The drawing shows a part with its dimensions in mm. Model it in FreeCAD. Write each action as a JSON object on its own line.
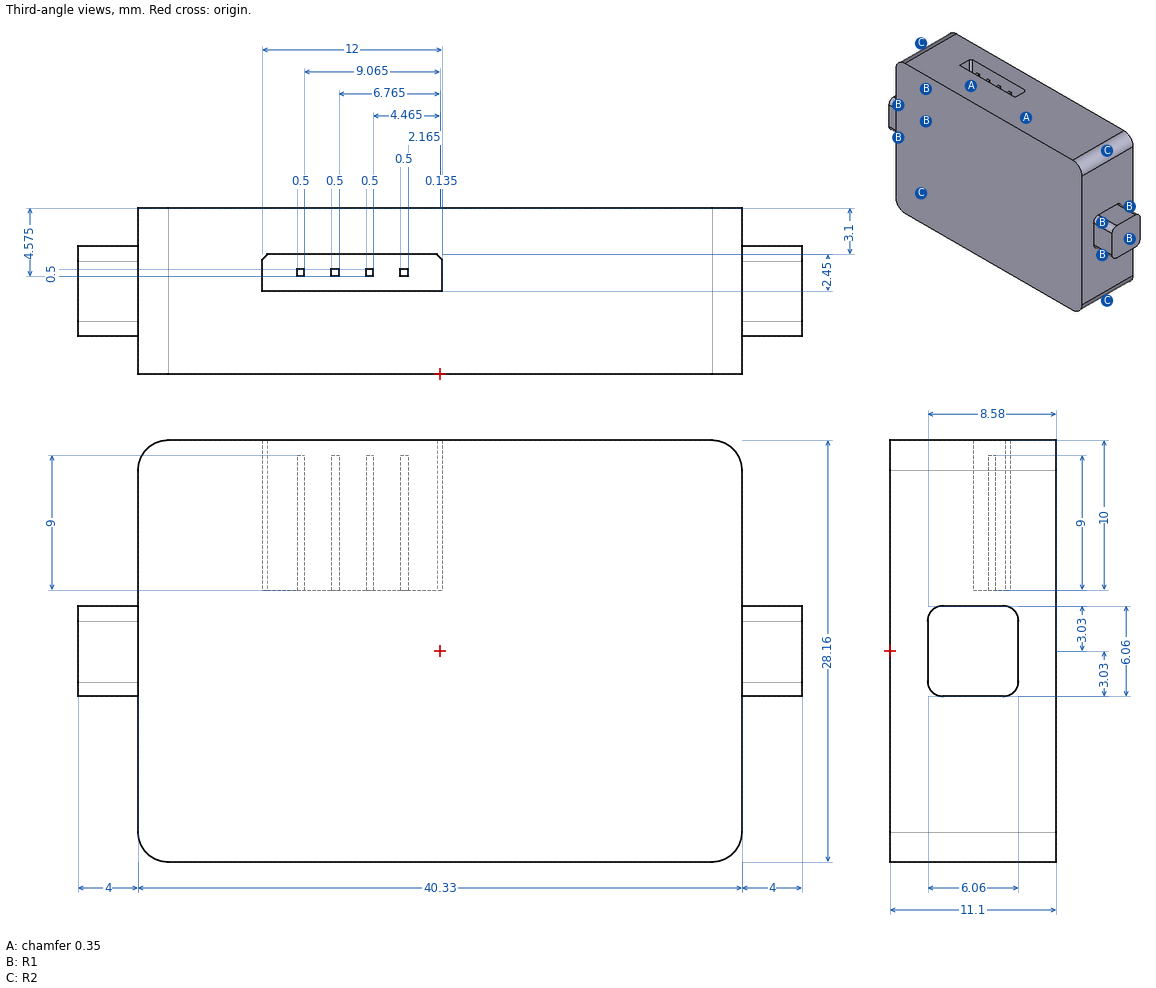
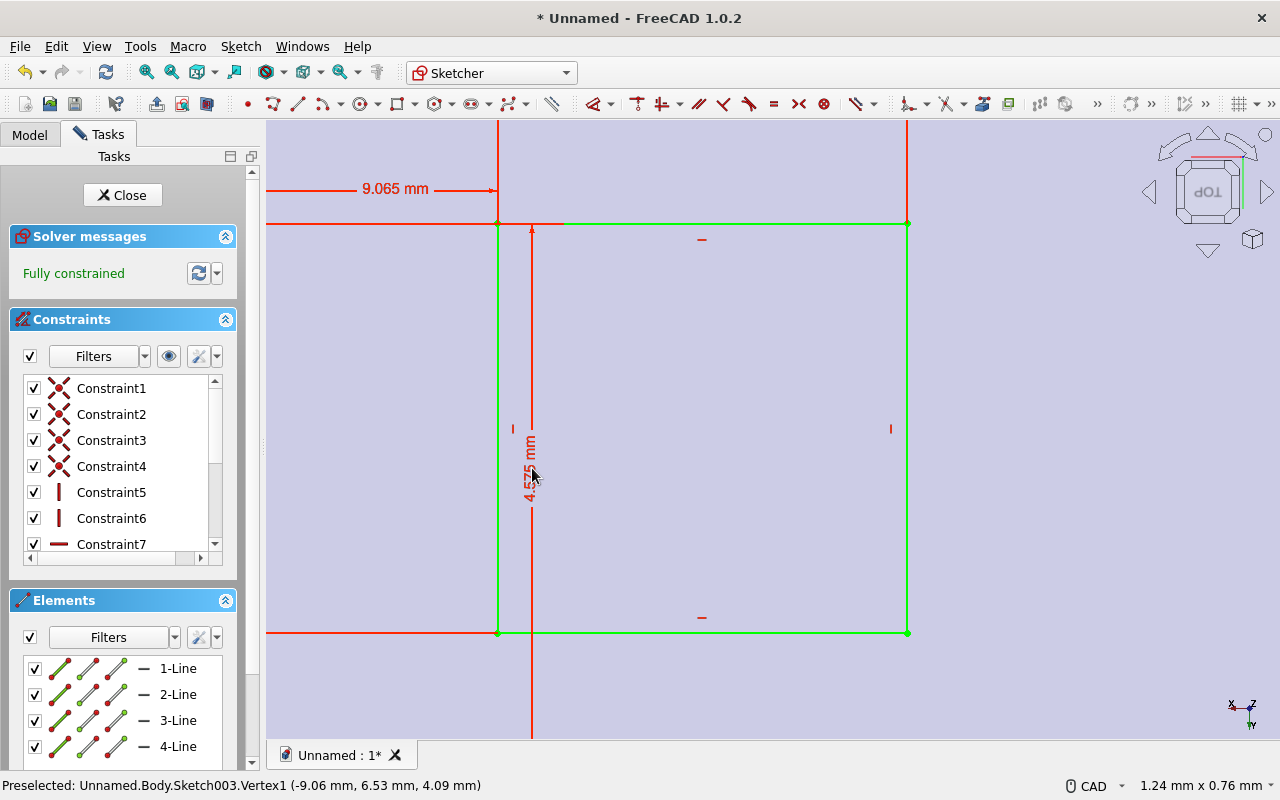
{"action": "left_click", "coordinate": [123, 195]}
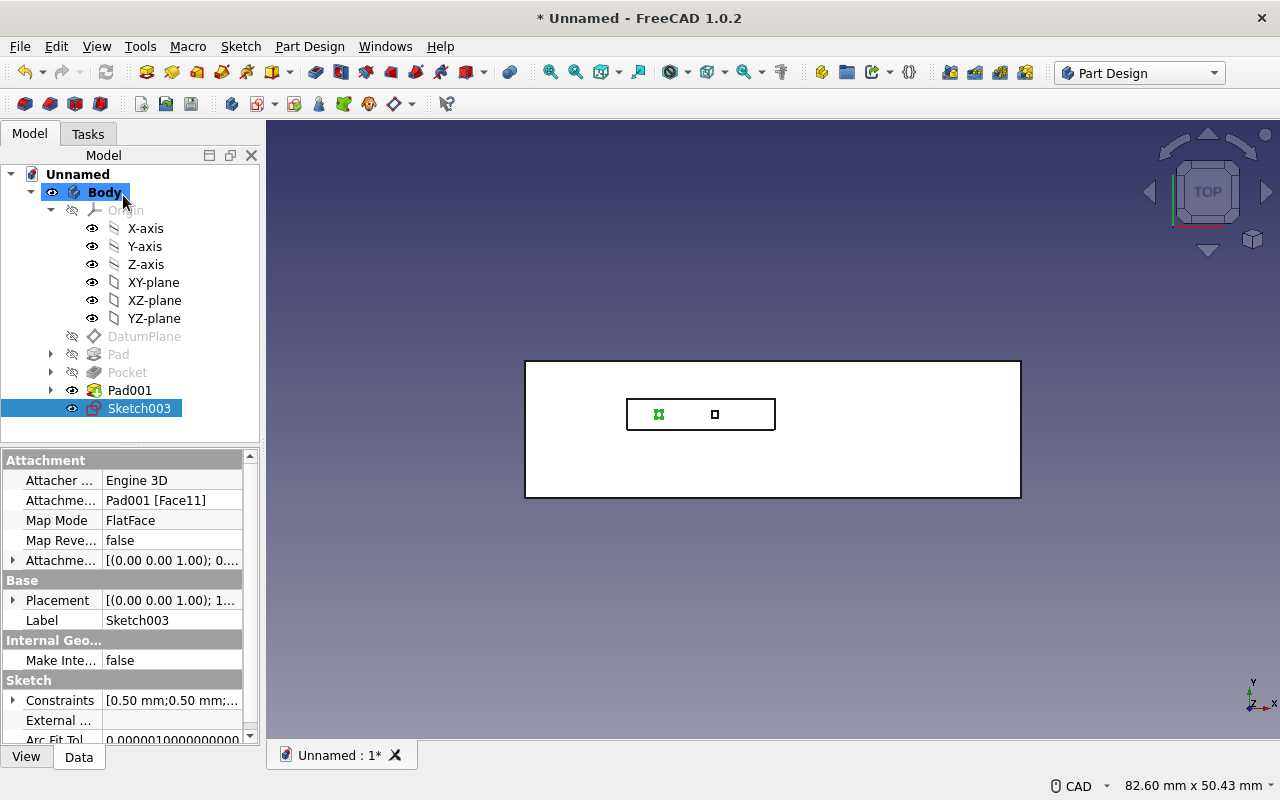
{"action": "left_click", "coordinate": [147, 72]}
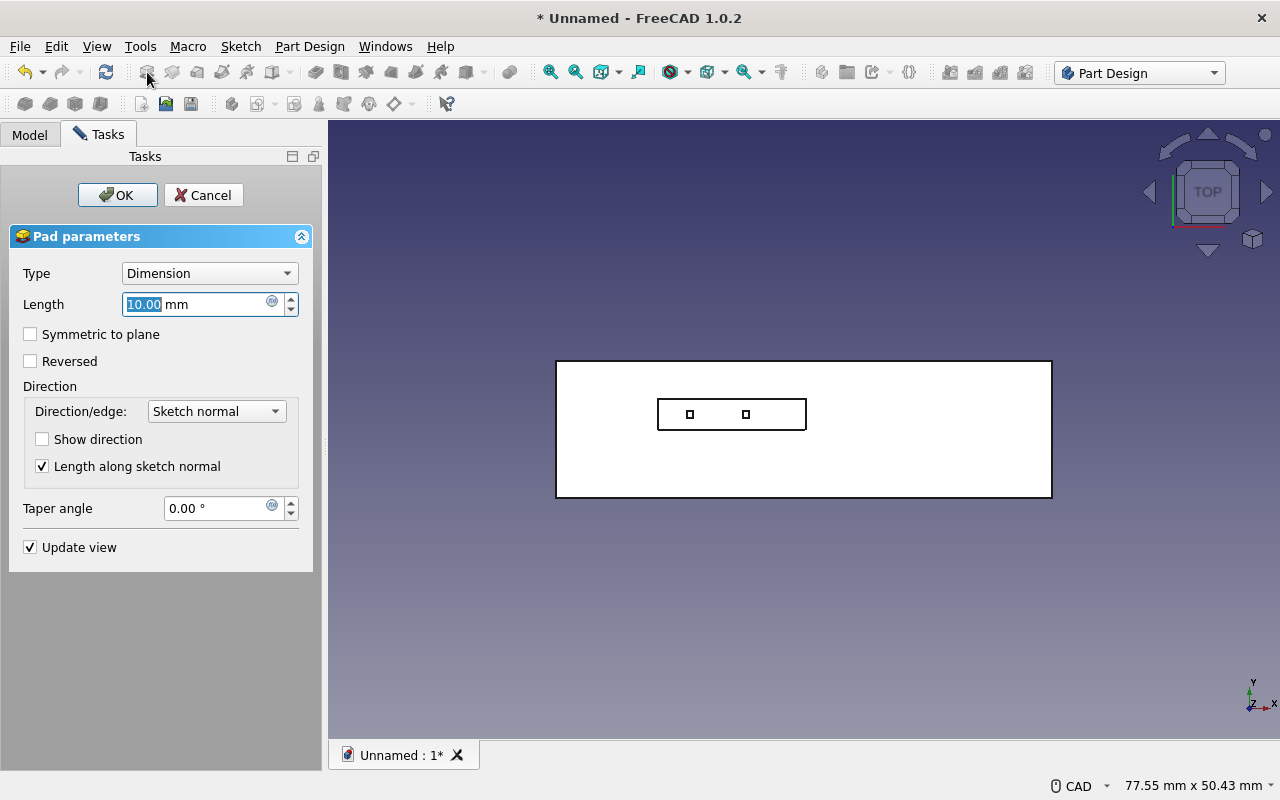
{"action": "type", "text": "9"}
{"action": "key", "text": "Tab"}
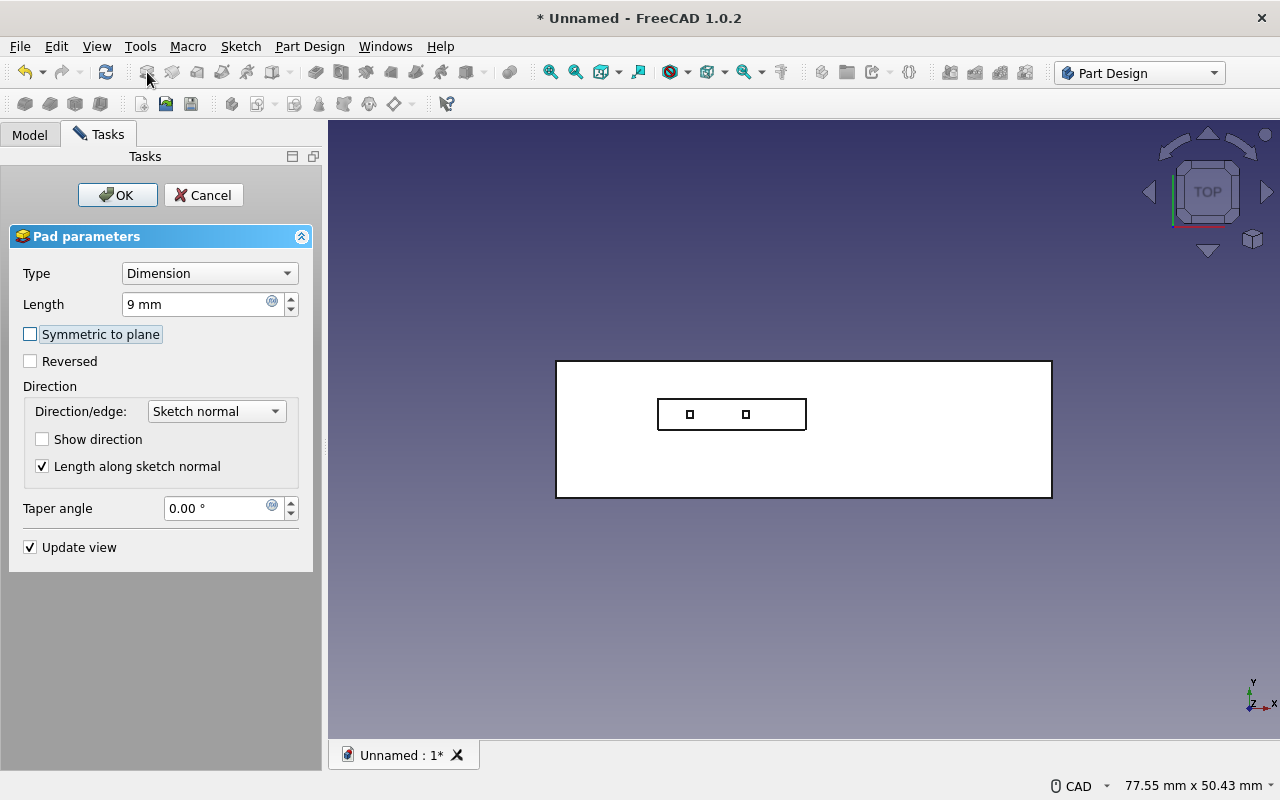
{"action": "left_click", "coordinate": [118, 195]}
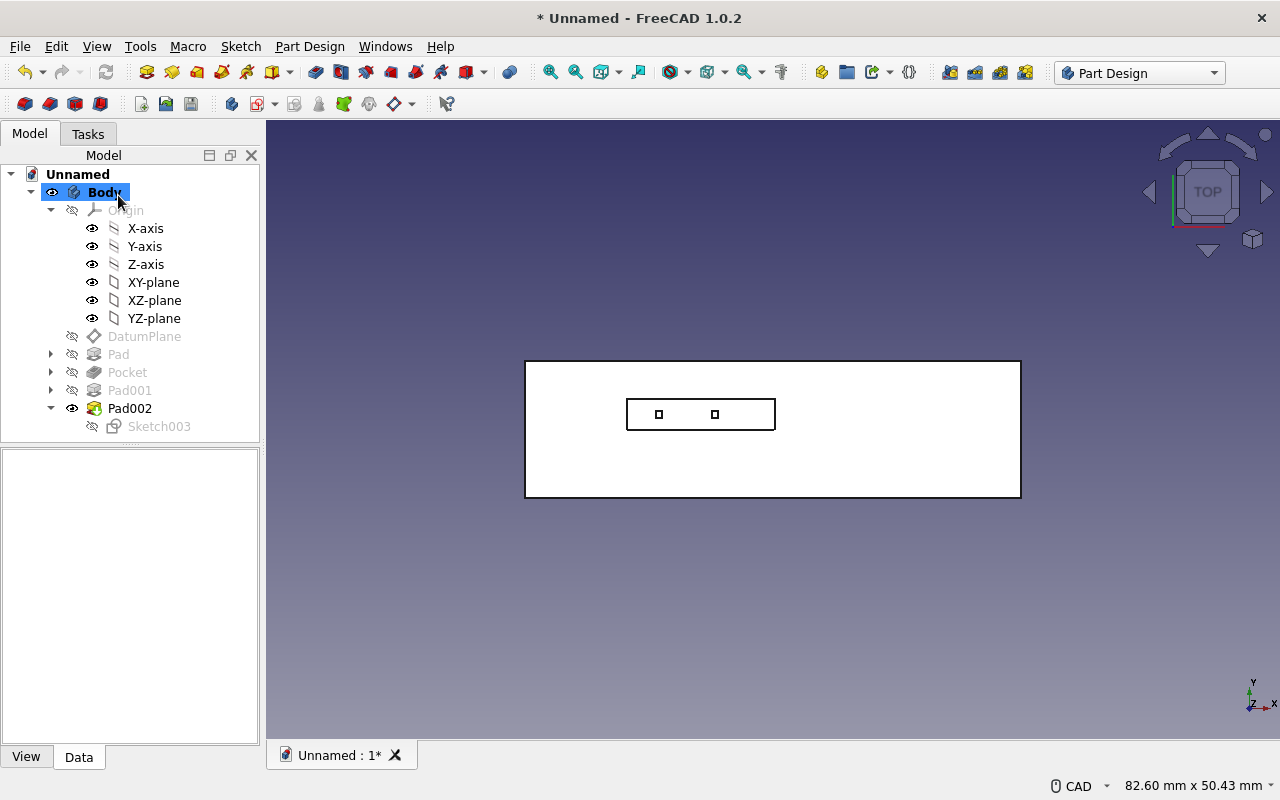
{"action": "left_click", "coordinate": [743, 413]}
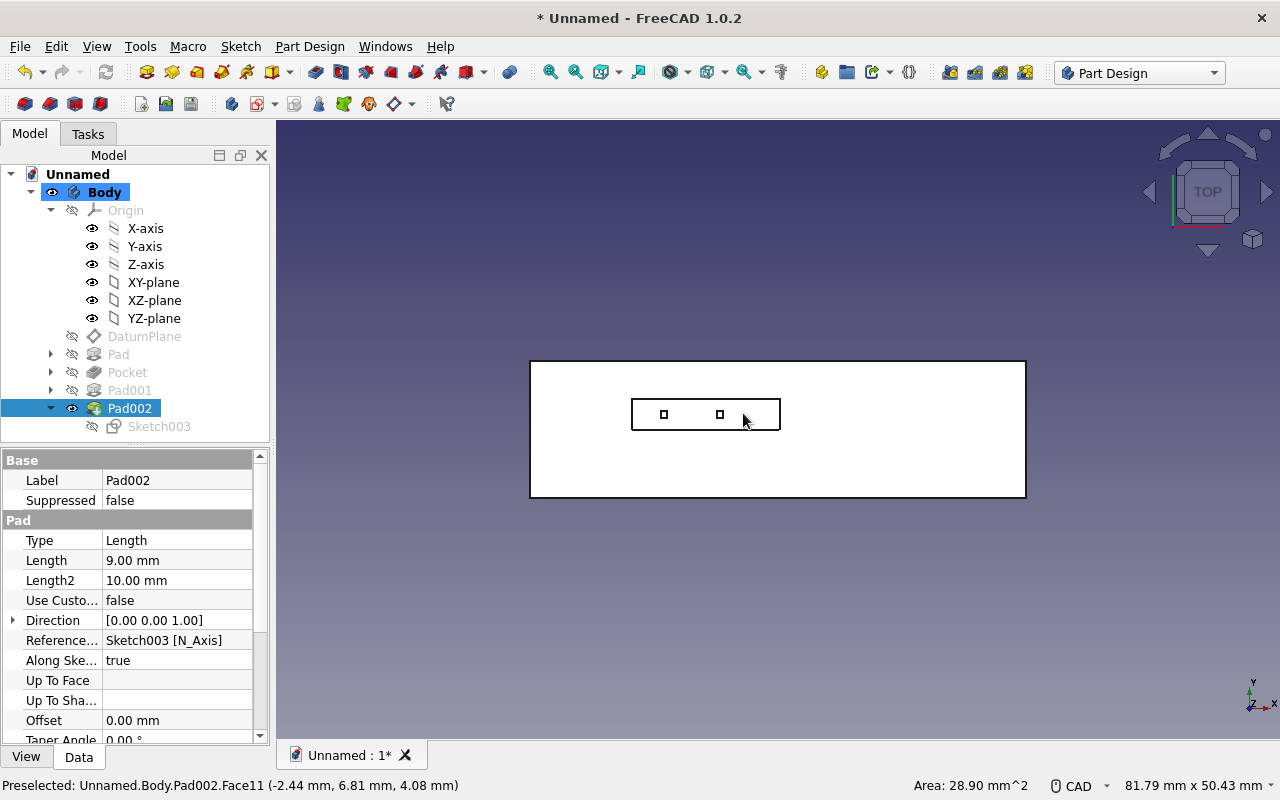
{"action": "left_click", "coordinate": [256, 104]}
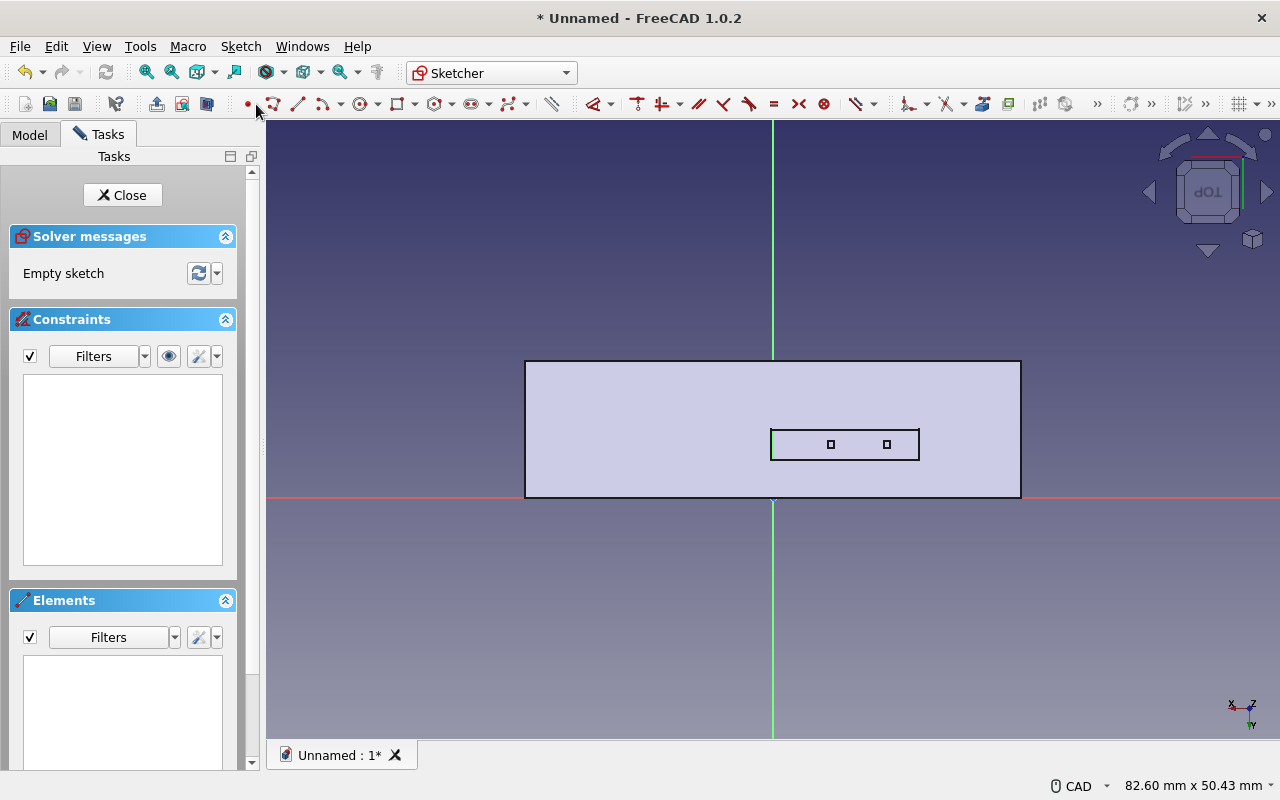
{"action": "left_click", "coordinate": [207, 104]}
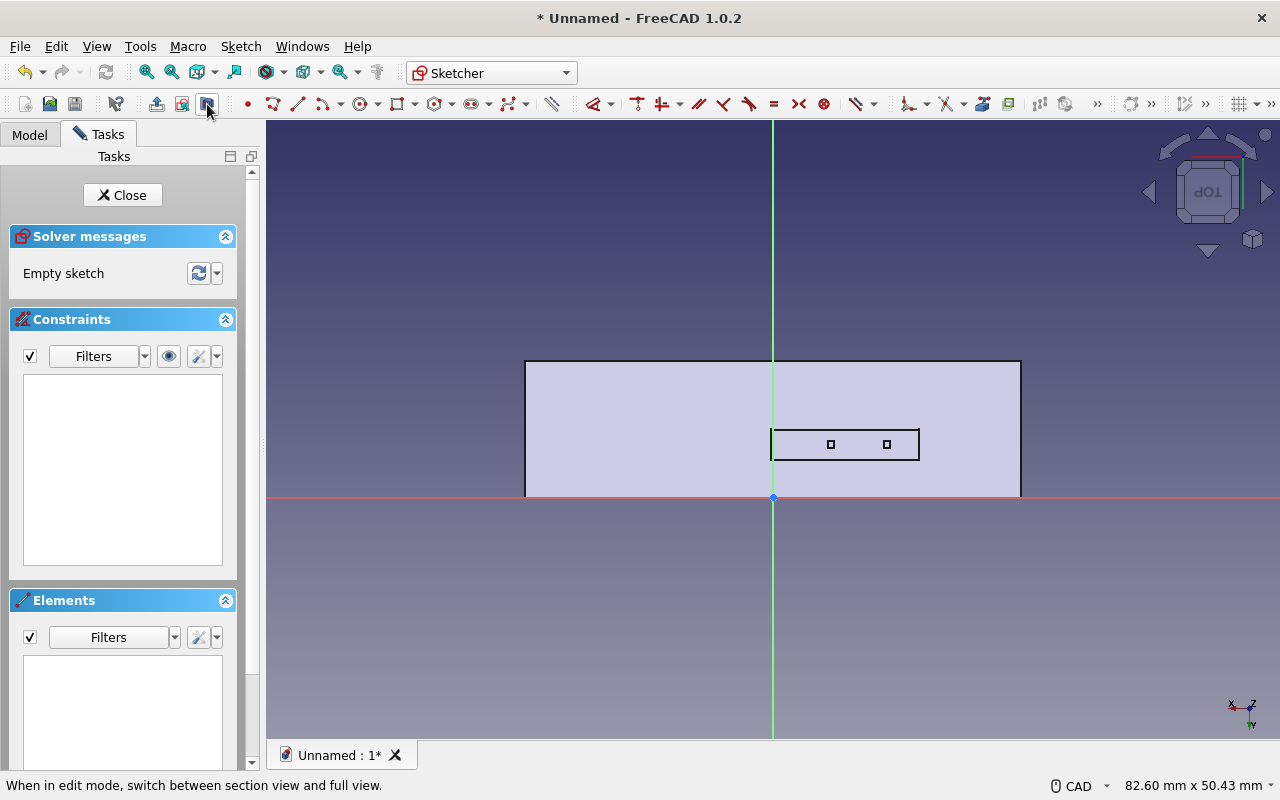
{"action": "scroll", "coordinate": [867, 445], "scroll_direction": "up", "scroll_amount": 15}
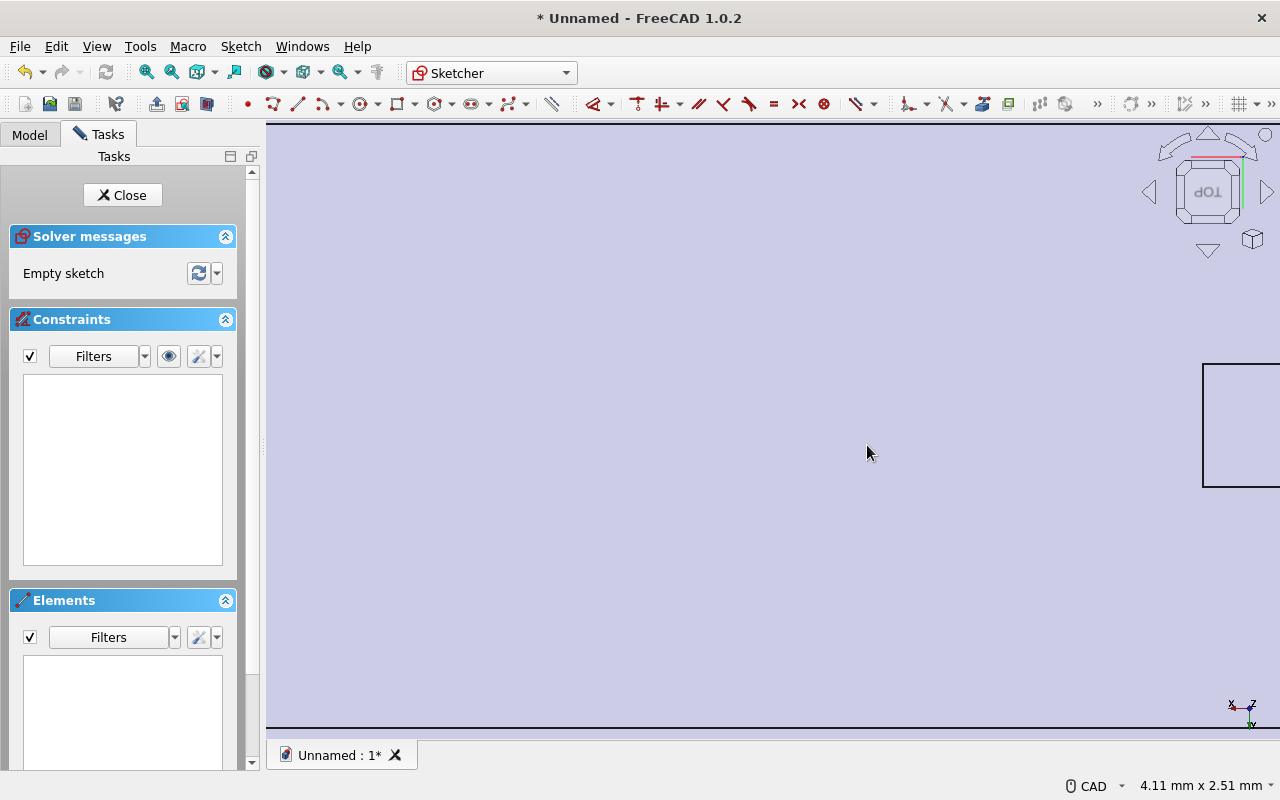
{"action": "scroll", "coordinate": [694, 424], "scroll_direction": "up", "scroll_amount": 6}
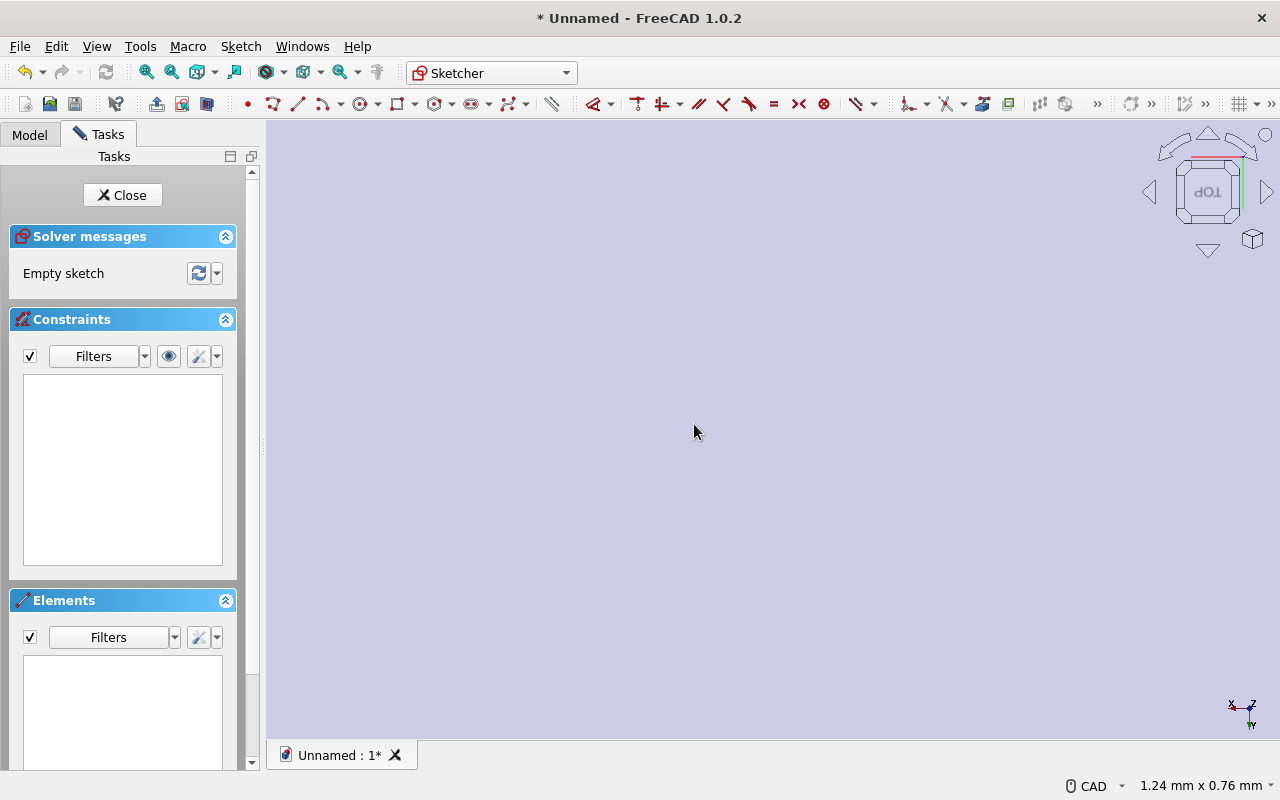
{"action": "left_click", "coordinate": [396, 104]}